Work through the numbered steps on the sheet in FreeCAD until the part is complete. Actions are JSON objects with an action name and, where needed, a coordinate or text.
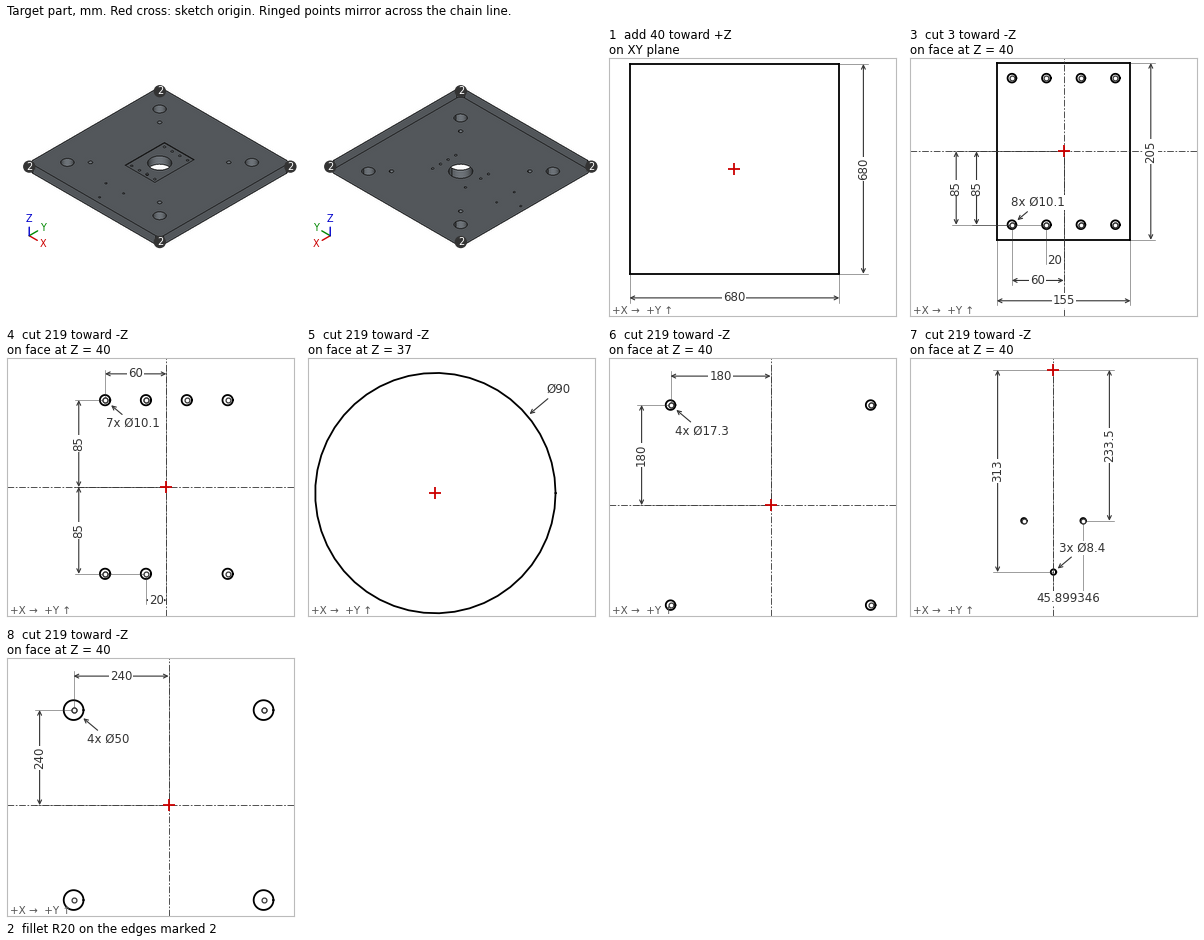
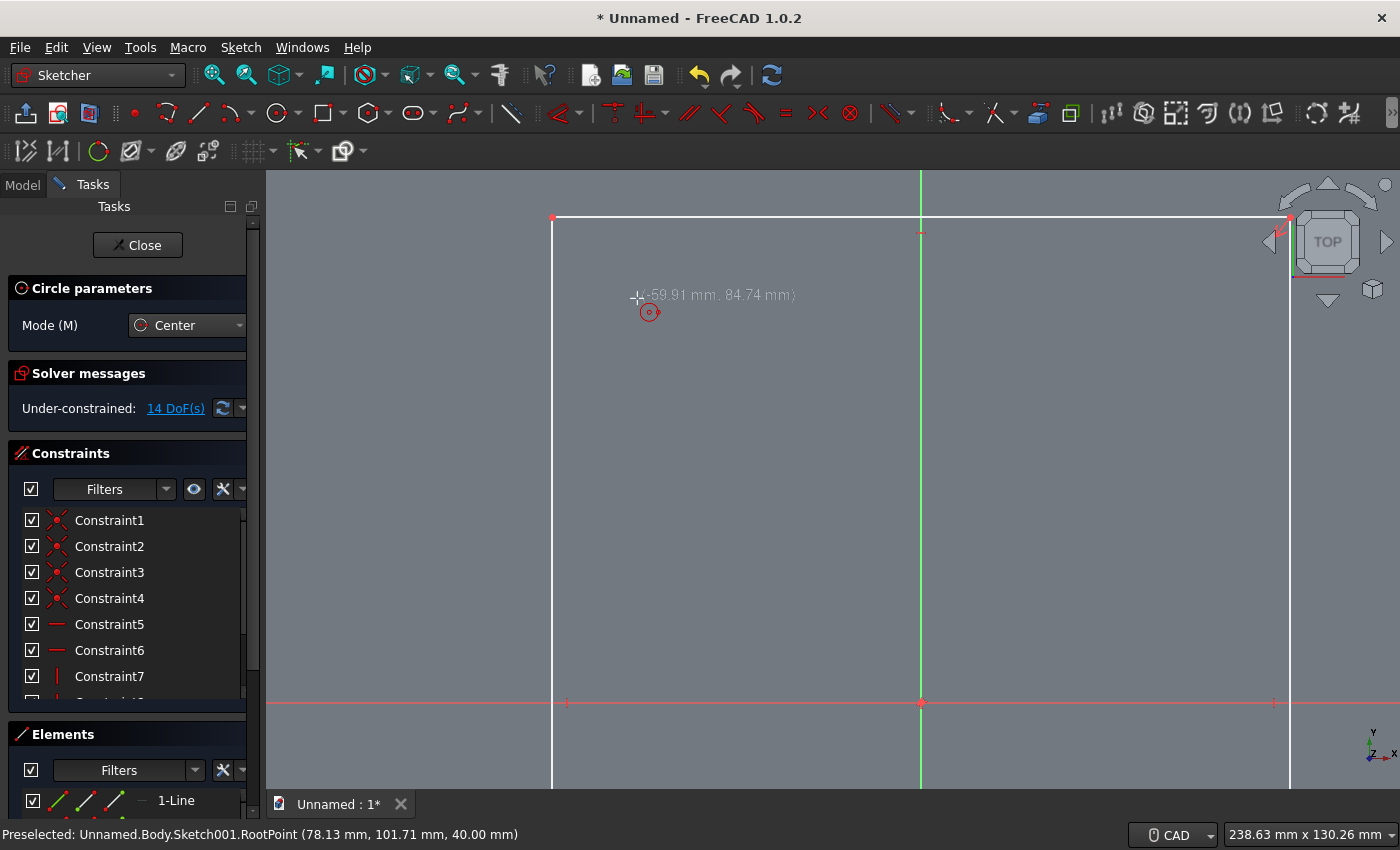
{"action": "left_click", "coordinate": [636, 299]}
{"action": "left_click", "coordinate": [653, 282]}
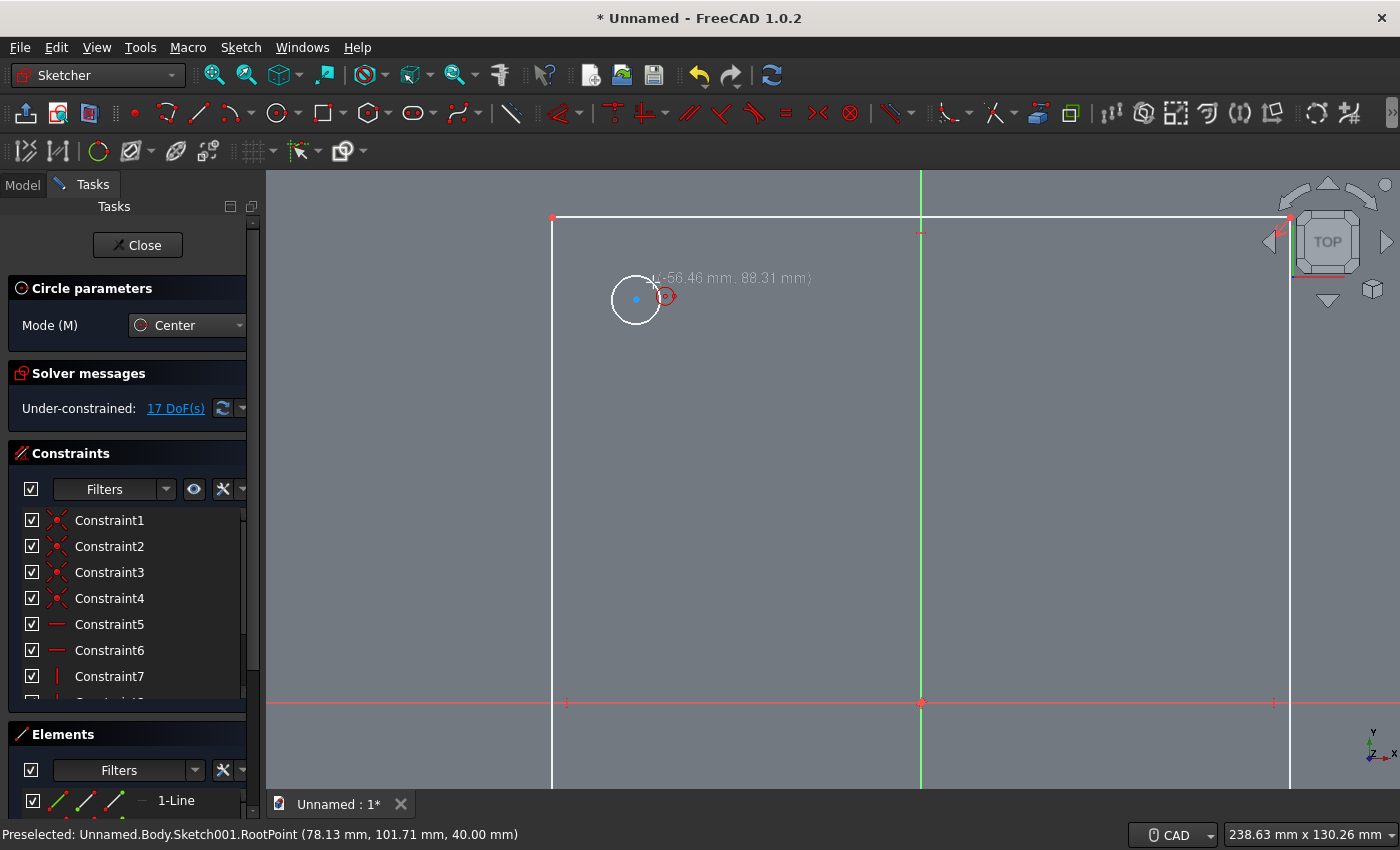
{"action": "left_click", "coordinate": [826, 299]}
{"action": "left_click", "coordinate": [843, 282]}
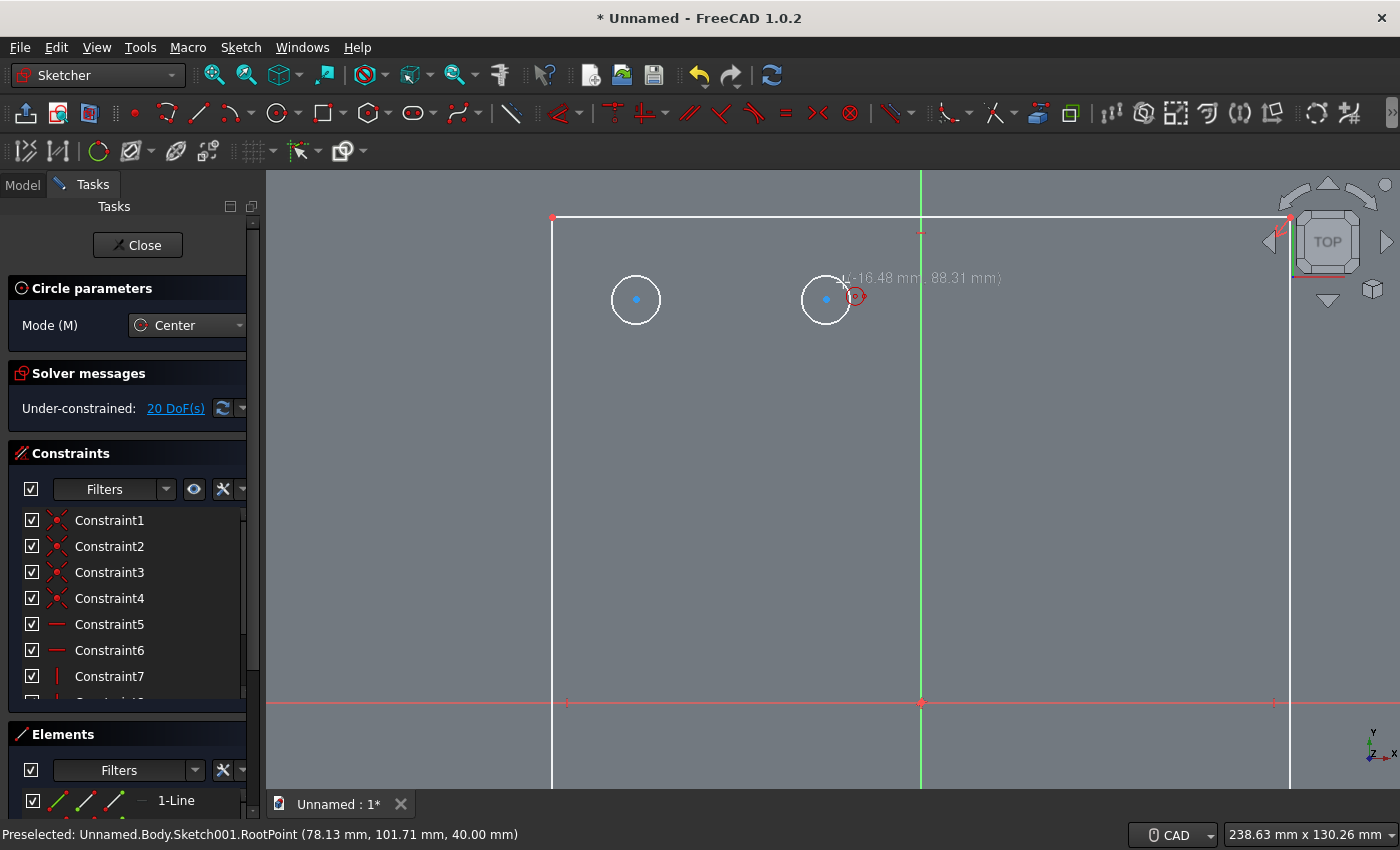
{"action": "left_click", "coordinate": [1016, 299]}
{"action": "left_click", "coordinate": [1033, 282]}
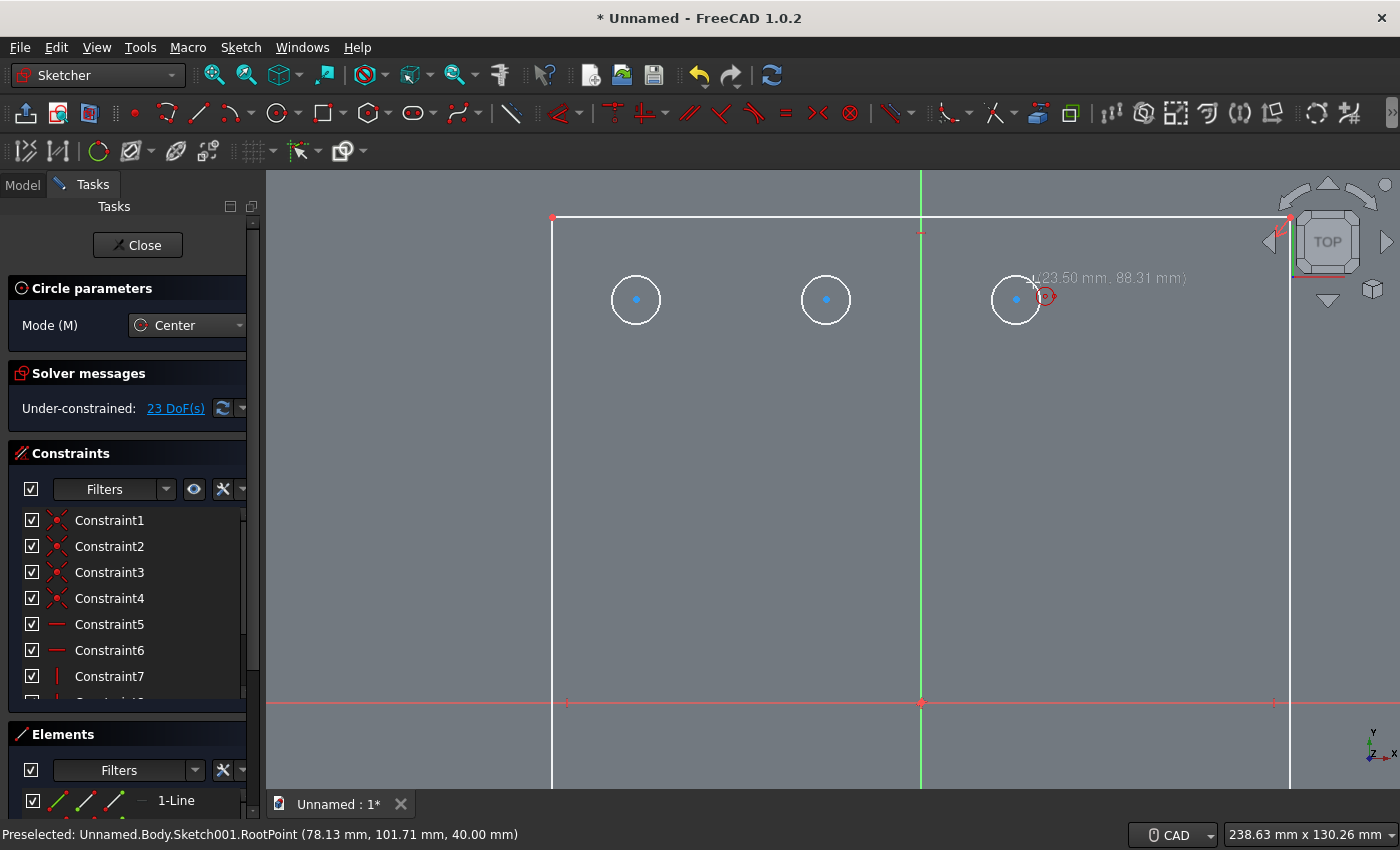
{"action": "left_click", "coordinate": [1206, 299]}
{"action": "left_click", "coordinate": [1223, 282]}
{"action": "key", "text": "Escape"}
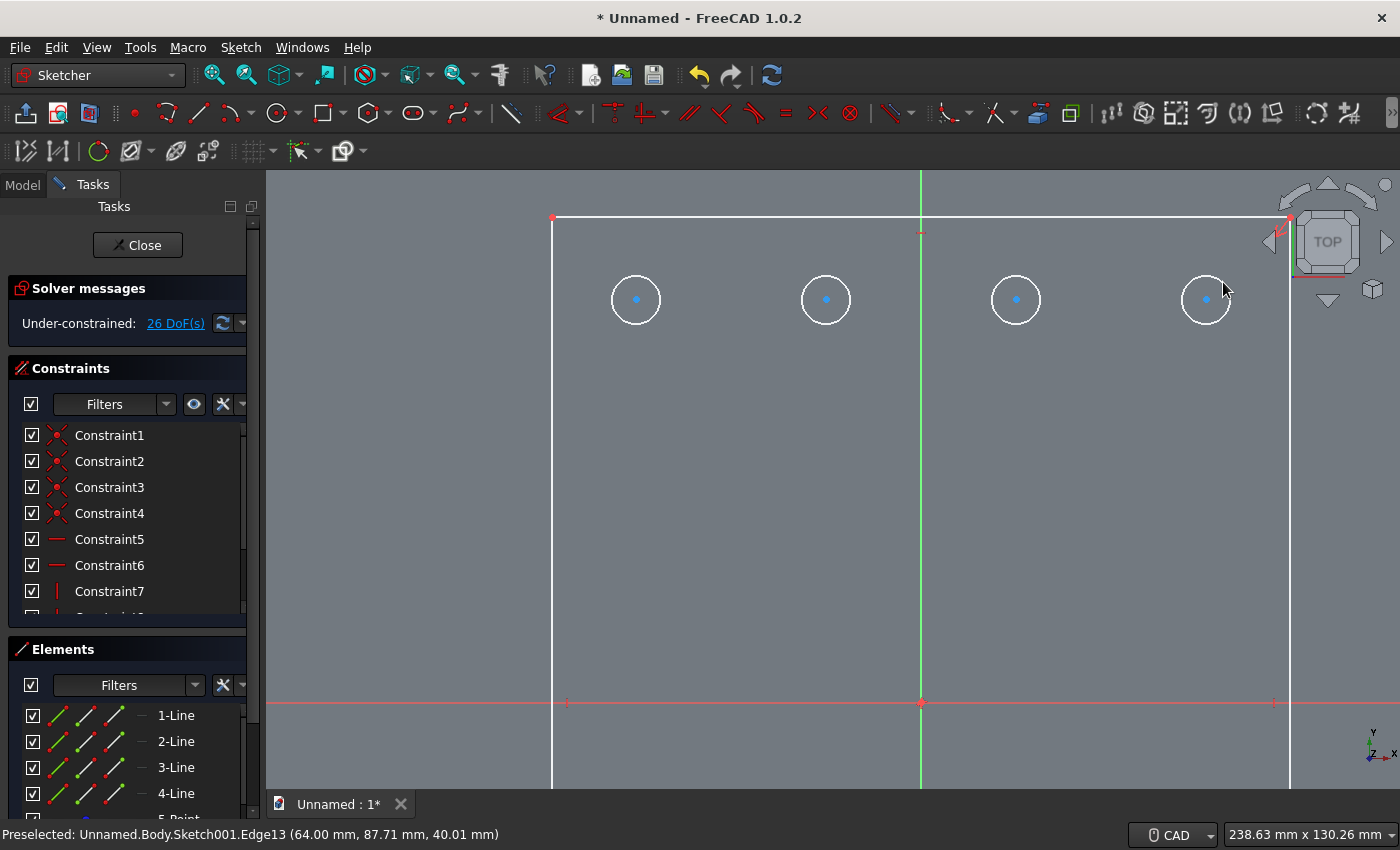
{"action": "scroll", "coordinate": [637, 297], "scroll_direction": "down", "scroll_amount": 4}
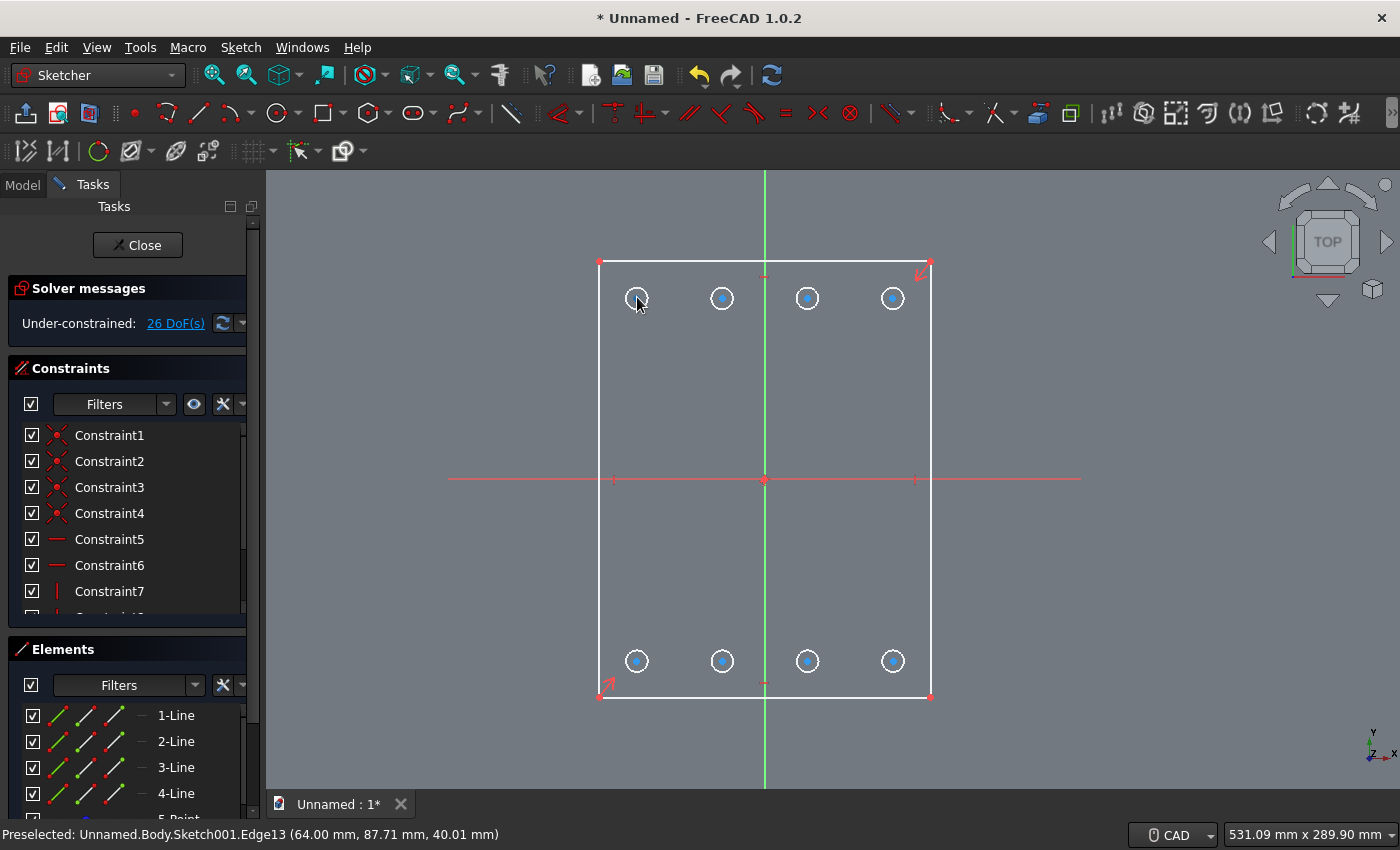
{"action": "scroll", "coordinate": [645, 654], "scroll_direction": "up", "scroll_amount": 2}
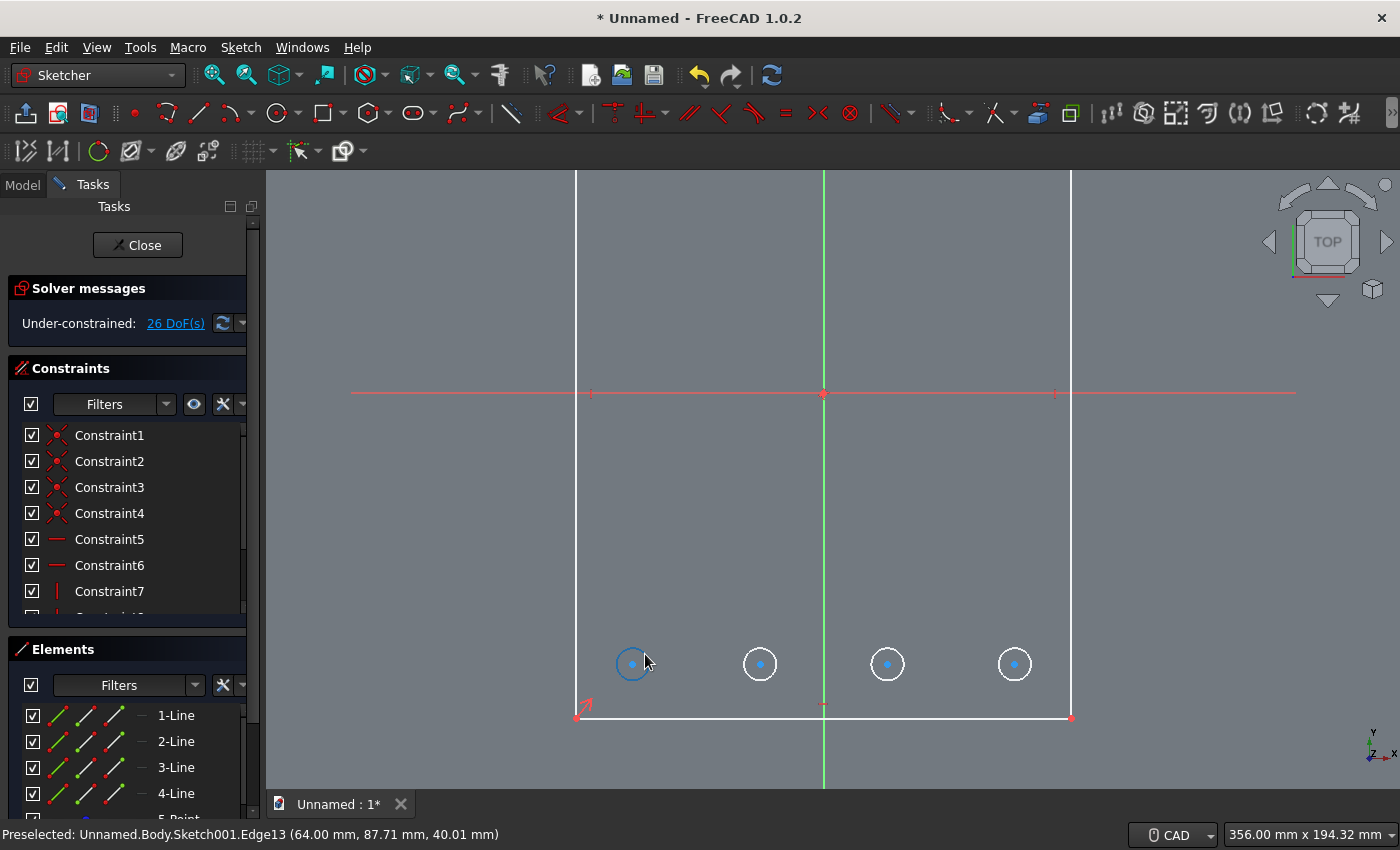
{"action": "left_click", "coordinate": [644, 653]}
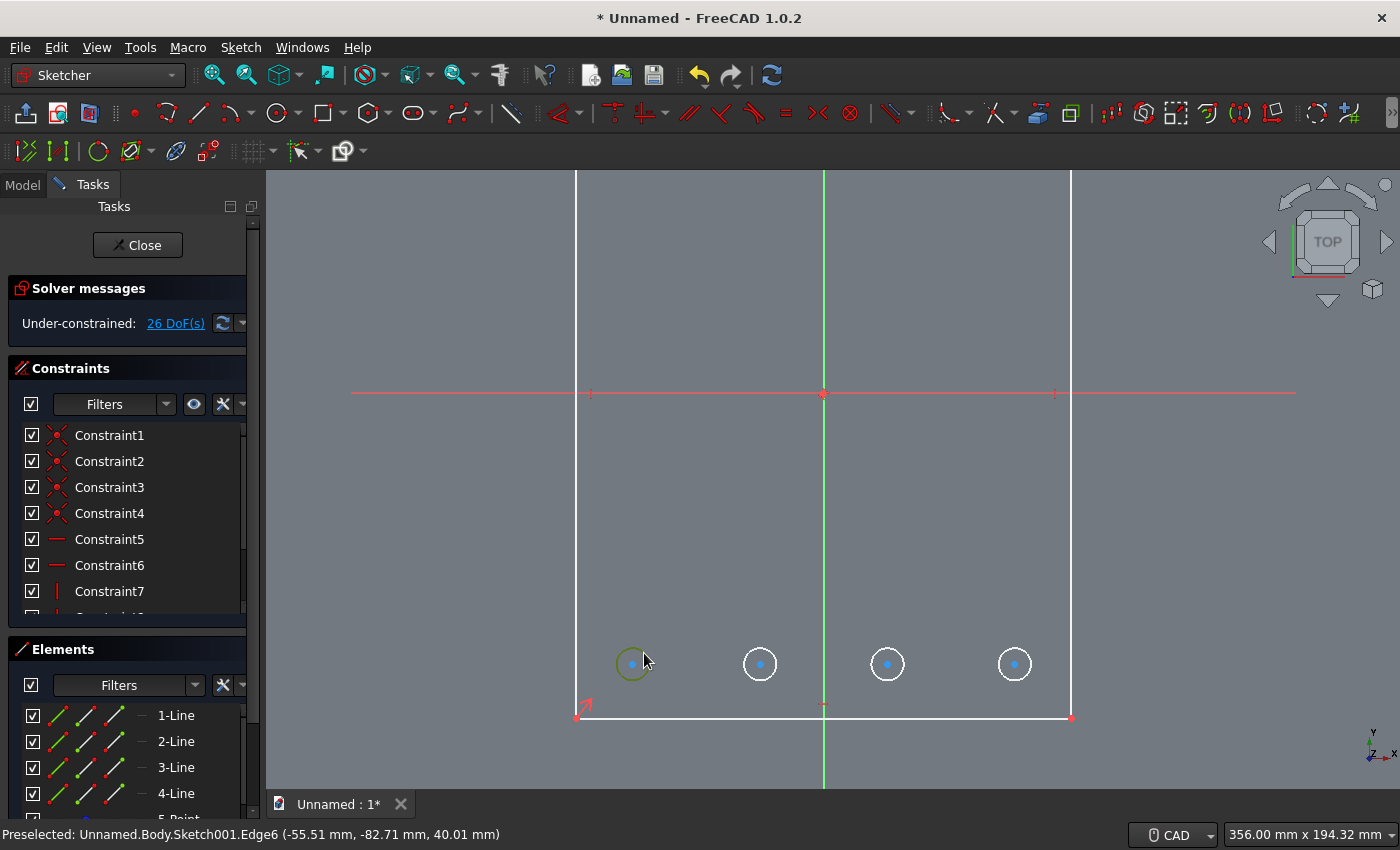
{"action": "left_click", "coordinate": [772, 653]}